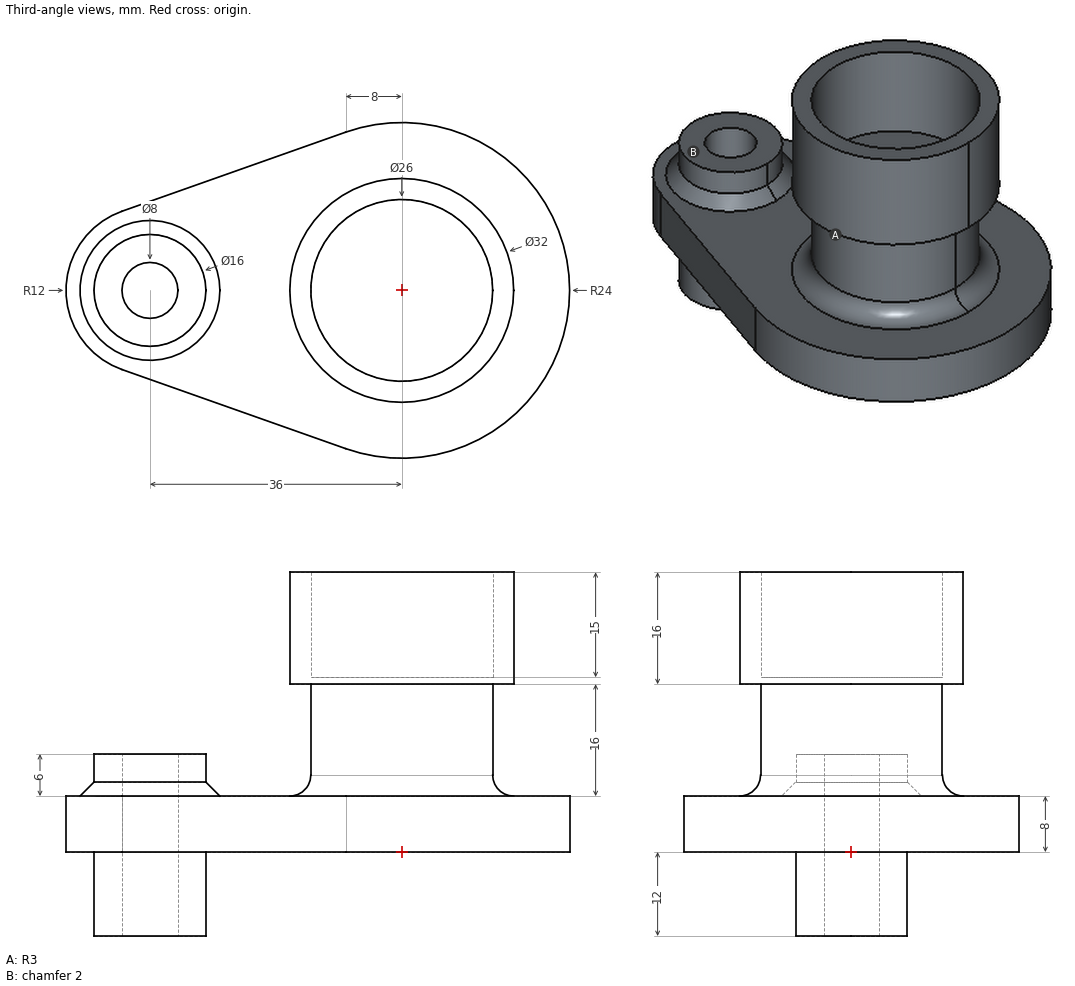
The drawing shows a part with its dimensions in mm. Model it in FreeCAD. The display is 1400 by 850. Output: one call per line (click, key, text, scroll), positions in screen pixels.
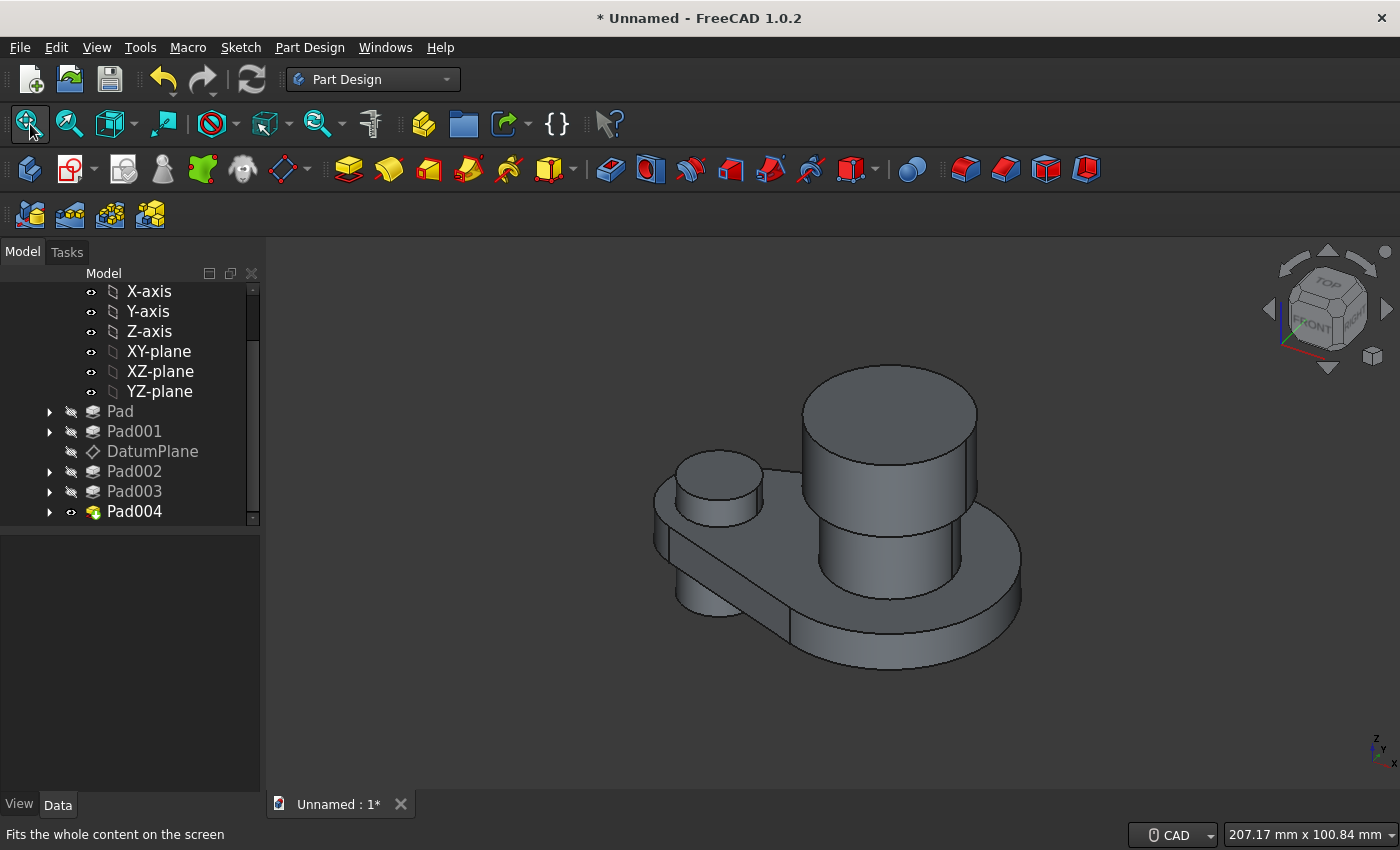
scroll(160, 407, down, 3)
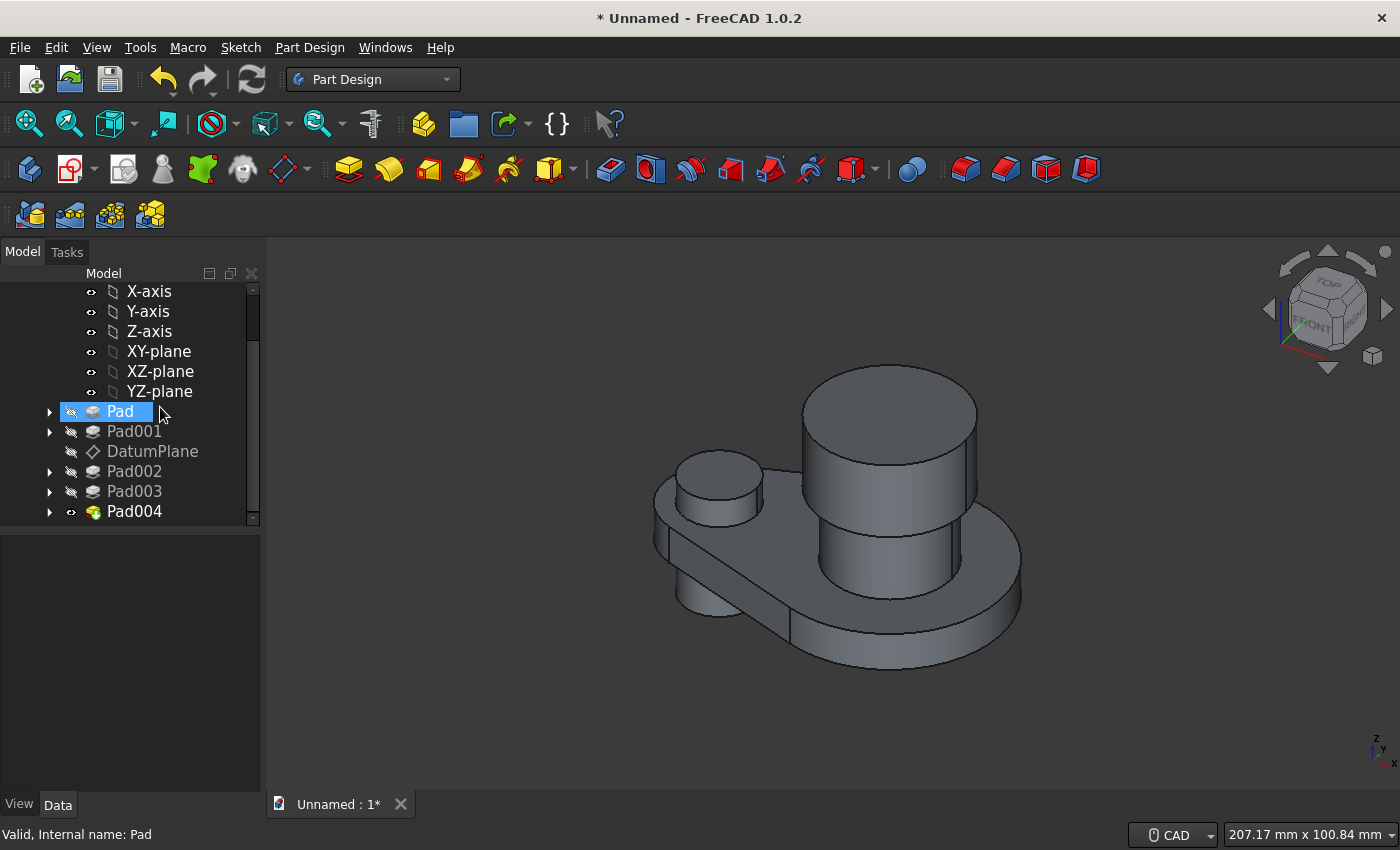
scroll(160, 407, up, 15)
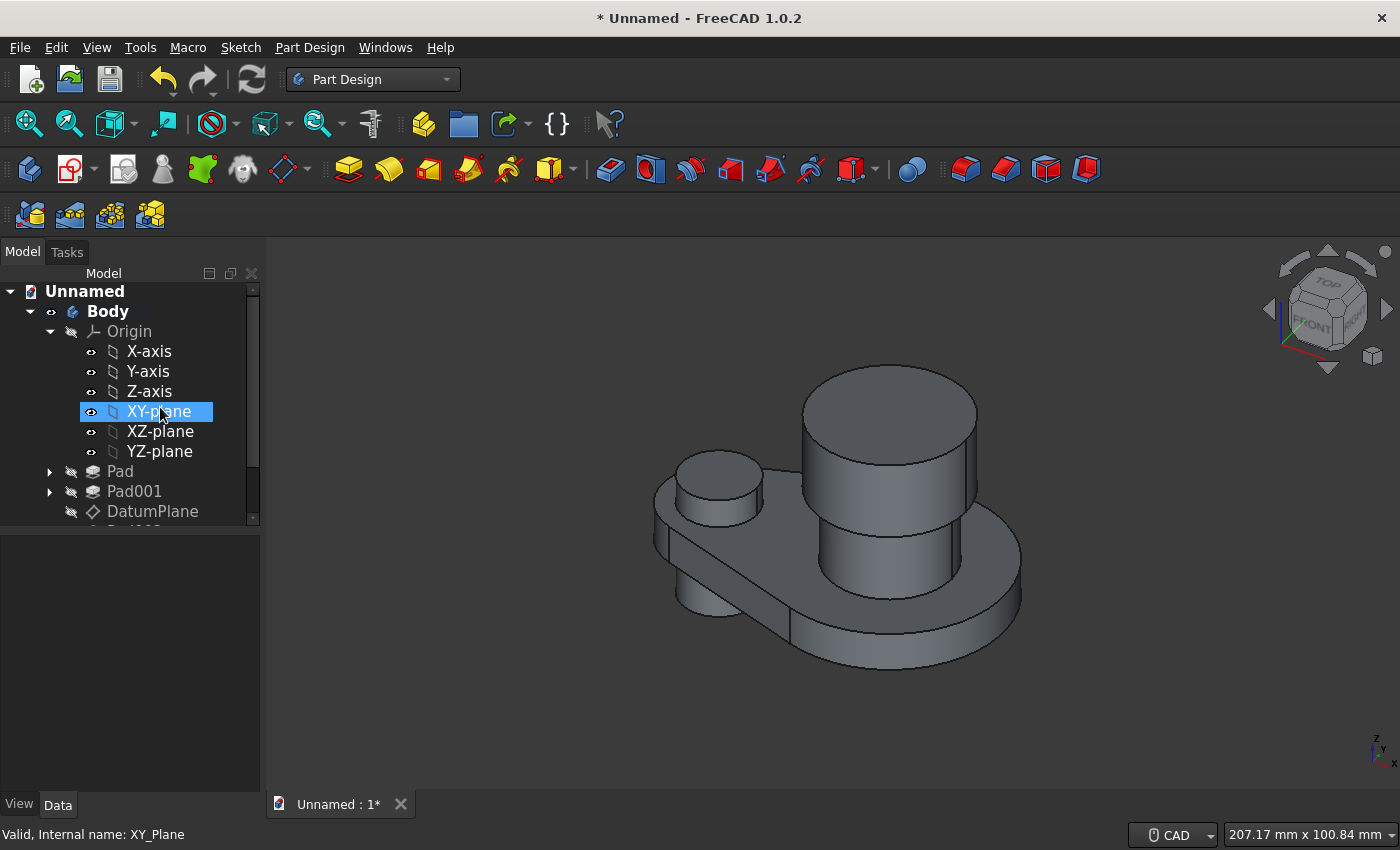
click(136, 412)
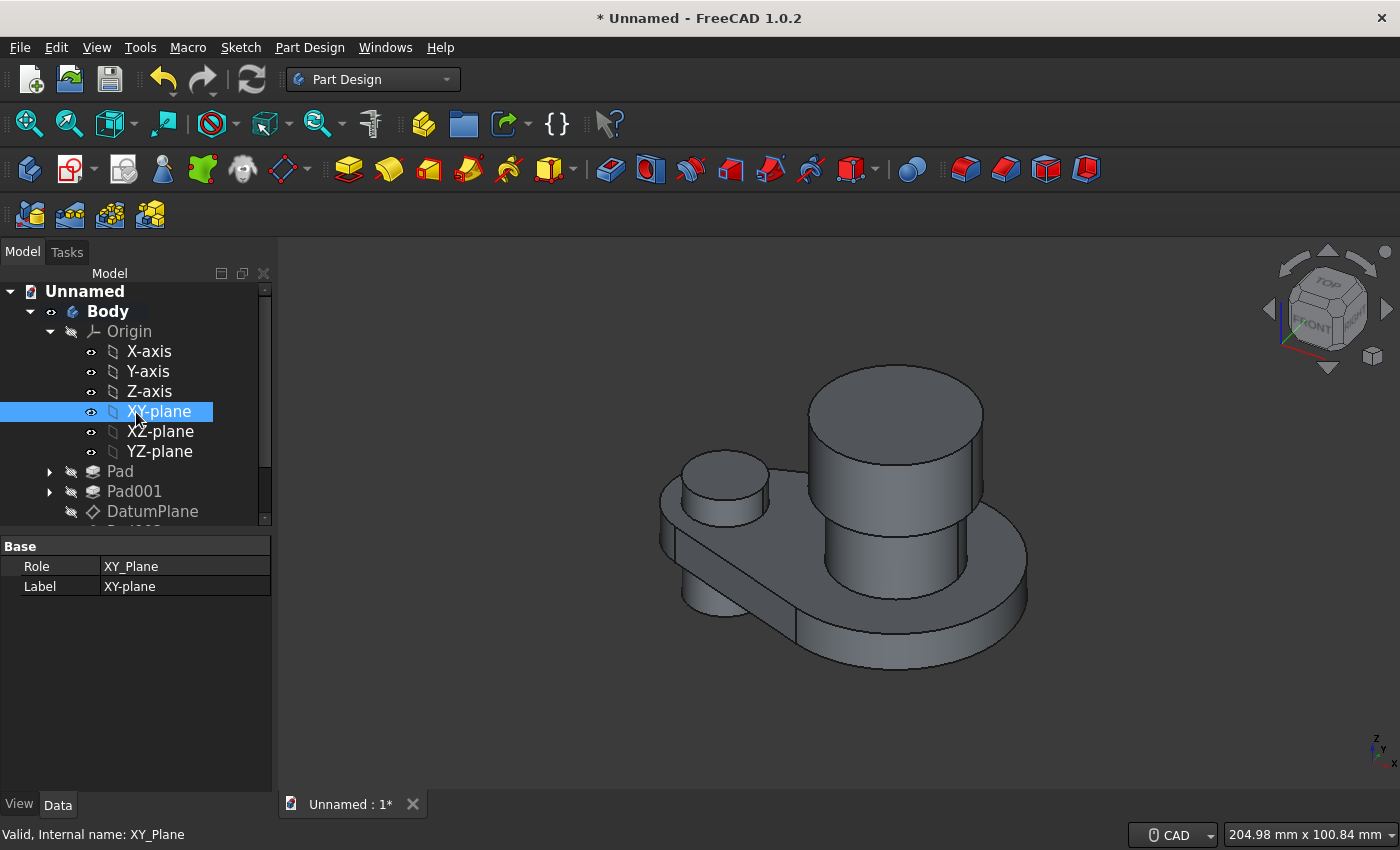
click(284, 170)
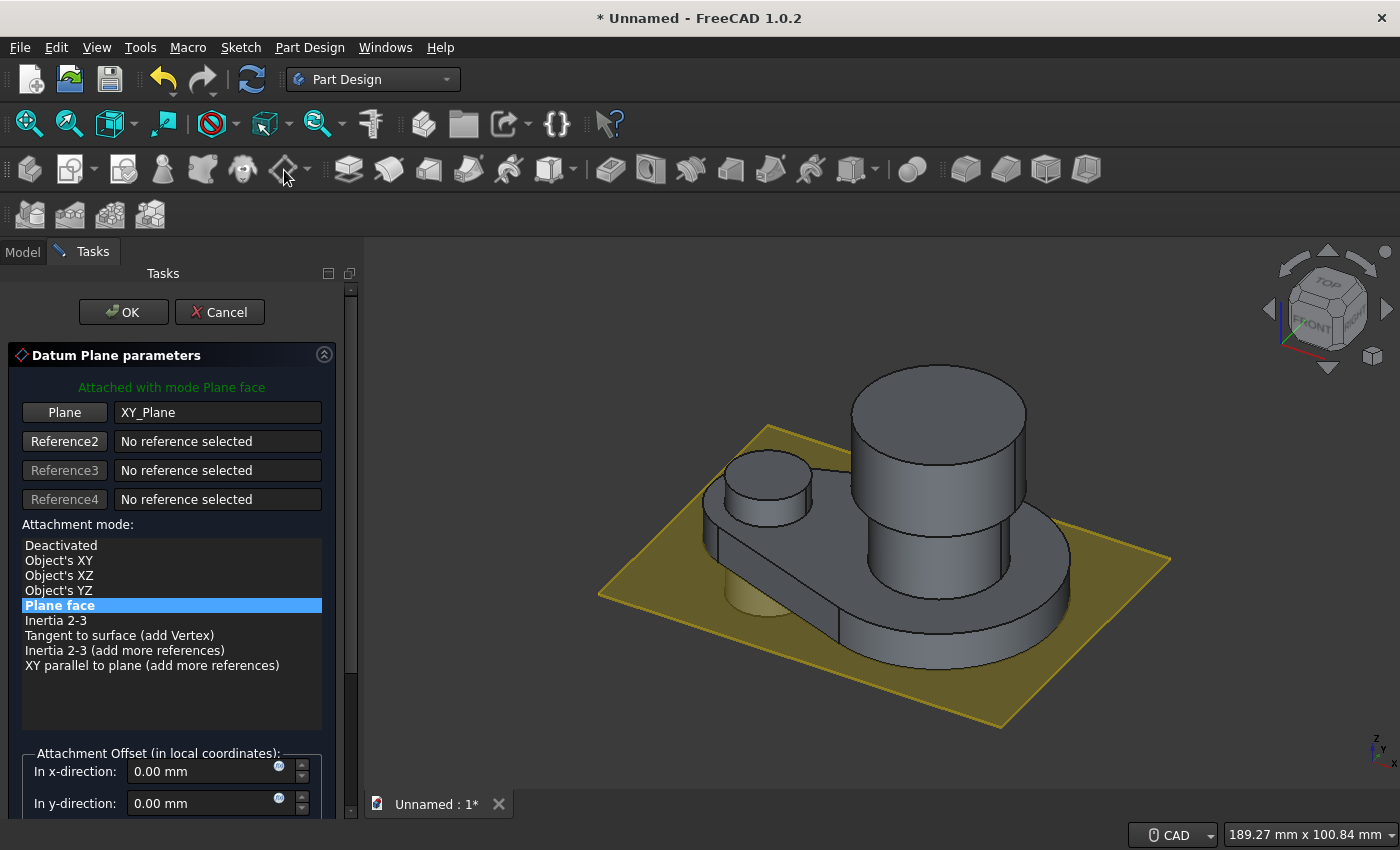
scroll(351, 550, down, 2)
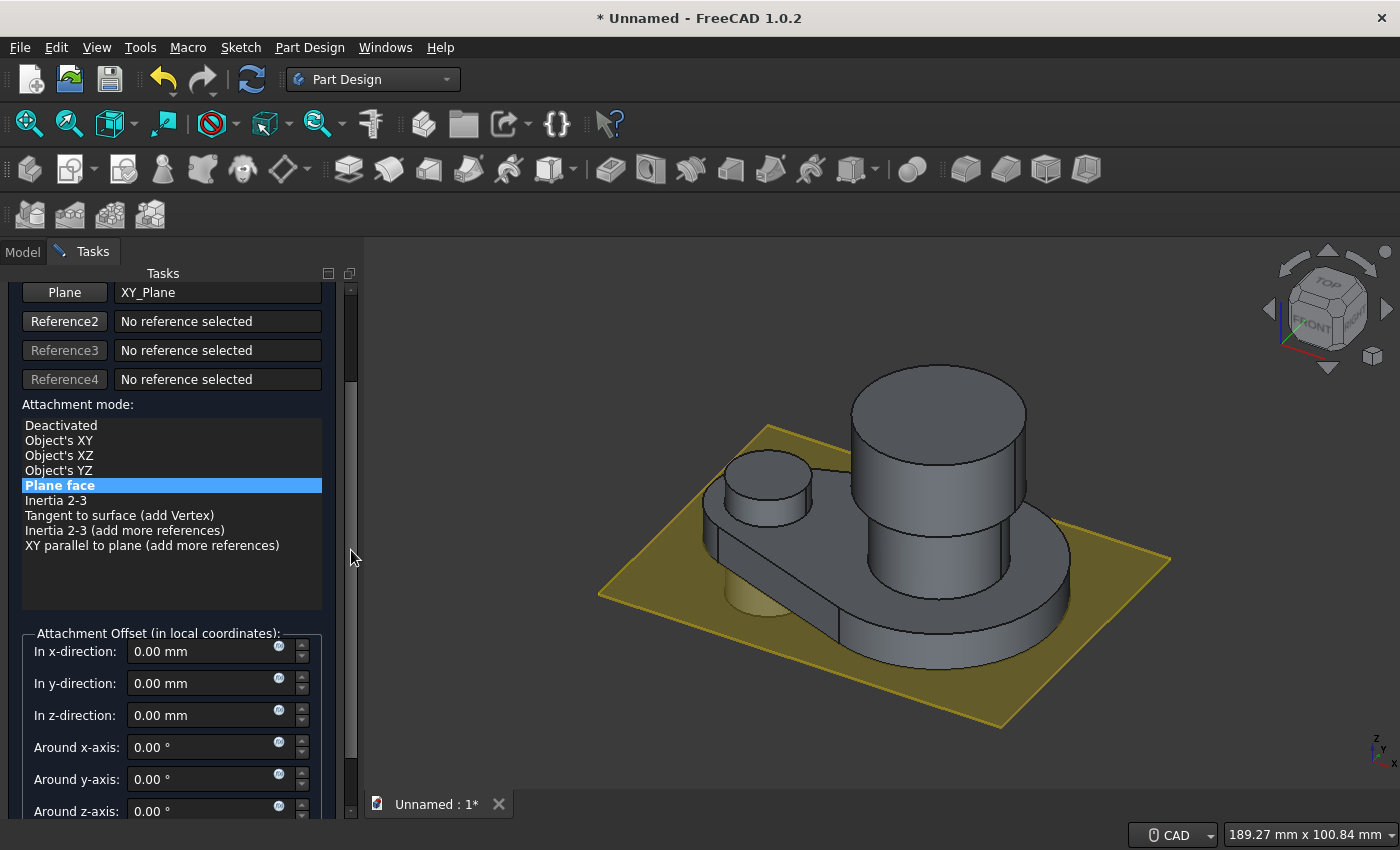
triple_click(210, 715)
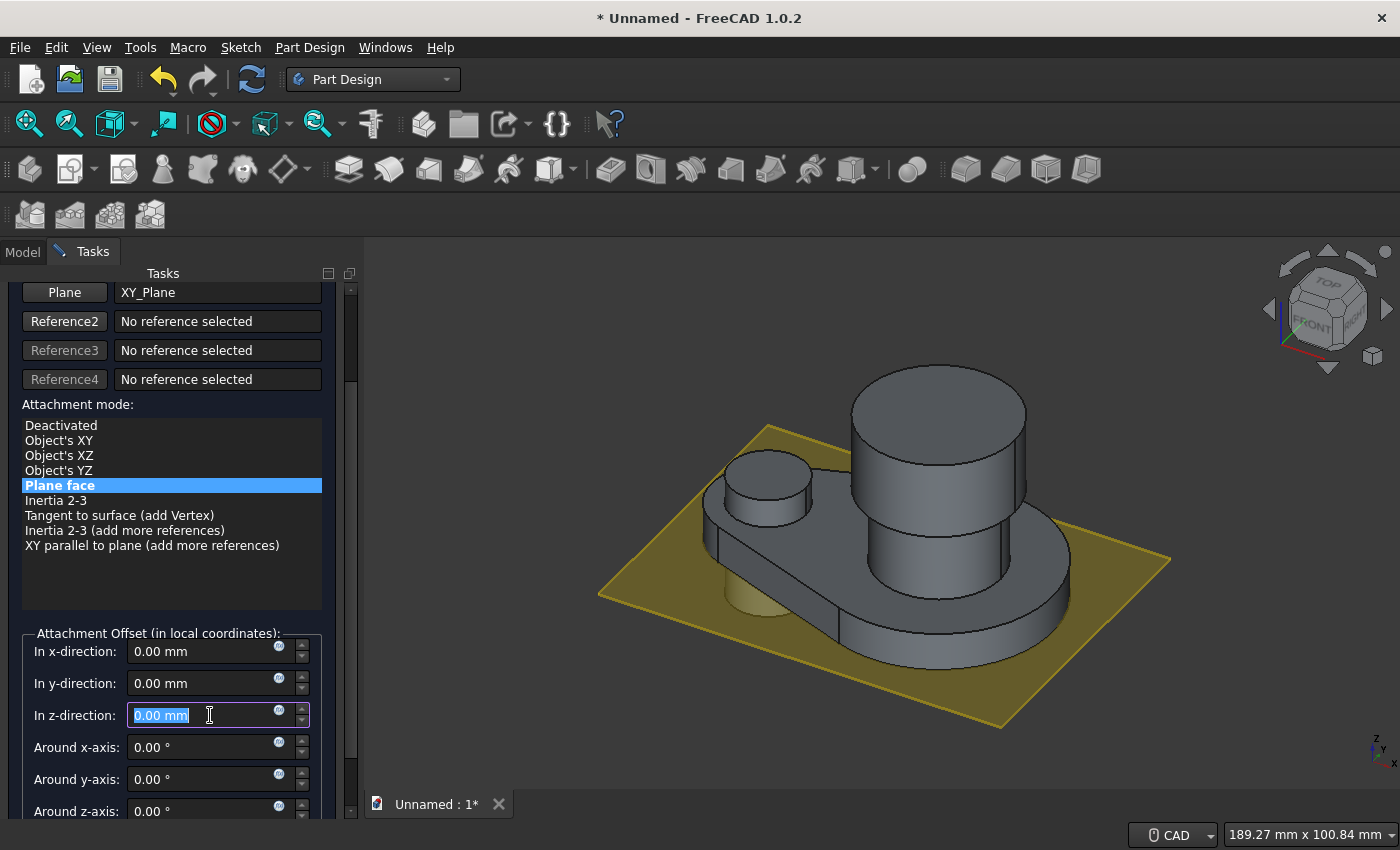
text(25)
key(Tab)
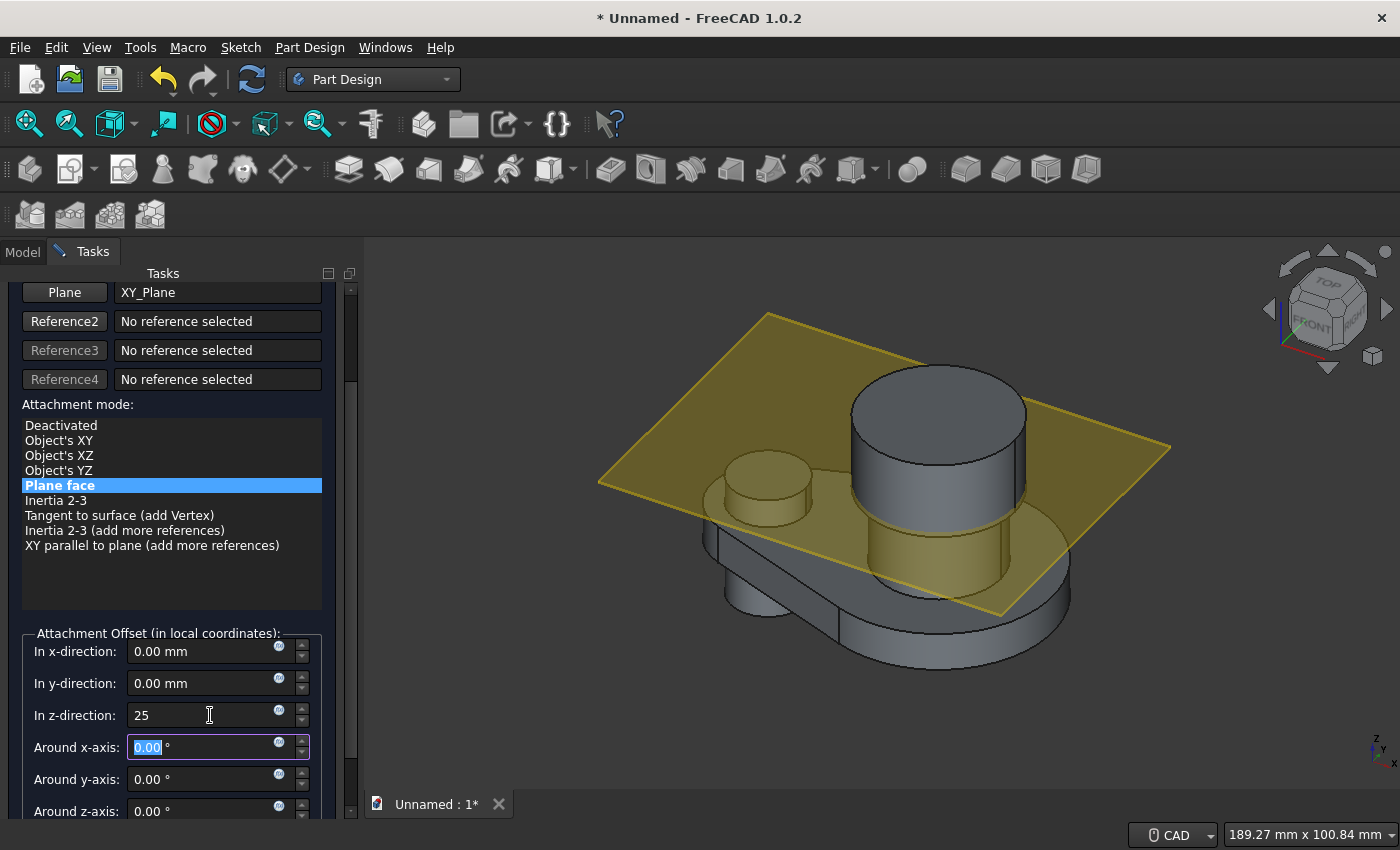
scroll(351, 550, up, 3)